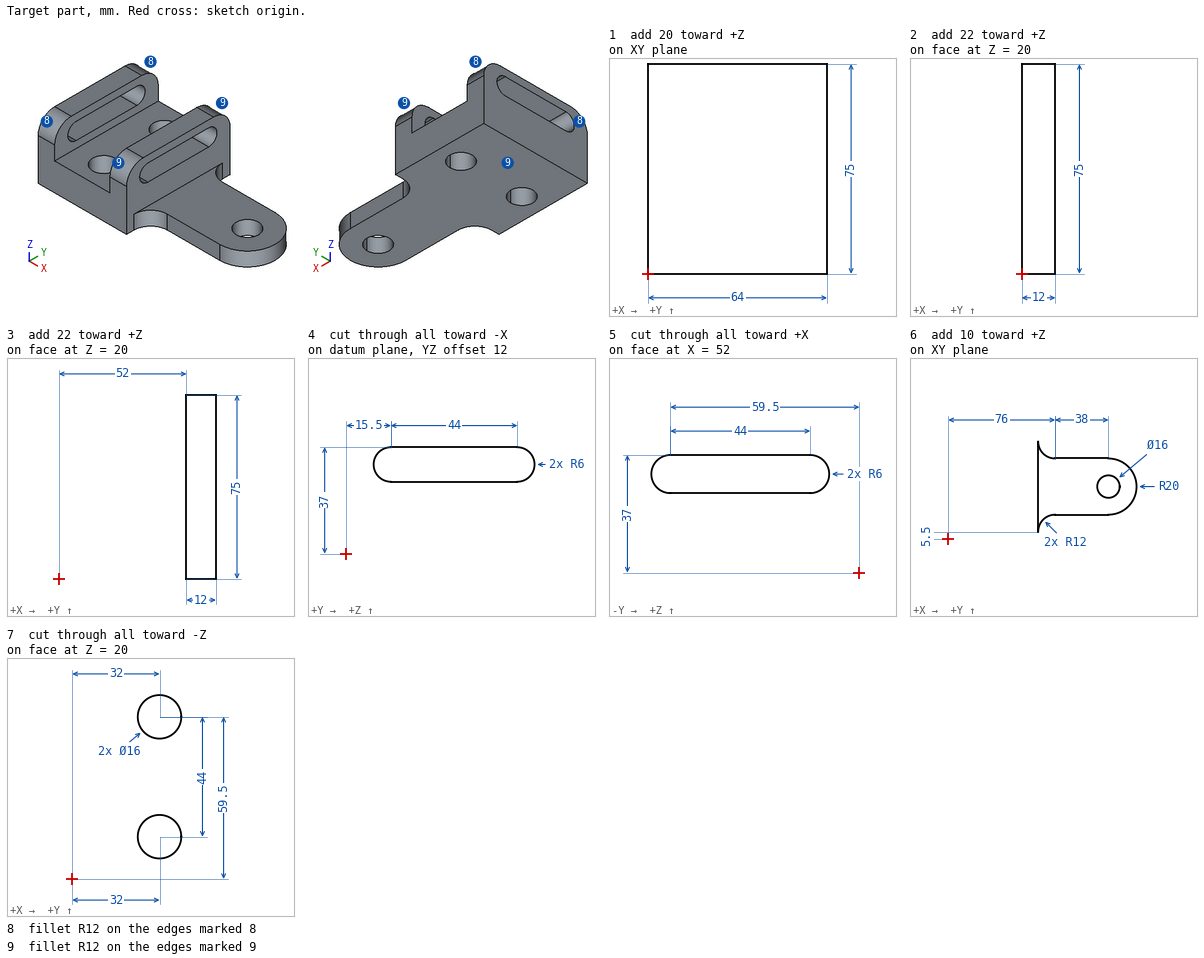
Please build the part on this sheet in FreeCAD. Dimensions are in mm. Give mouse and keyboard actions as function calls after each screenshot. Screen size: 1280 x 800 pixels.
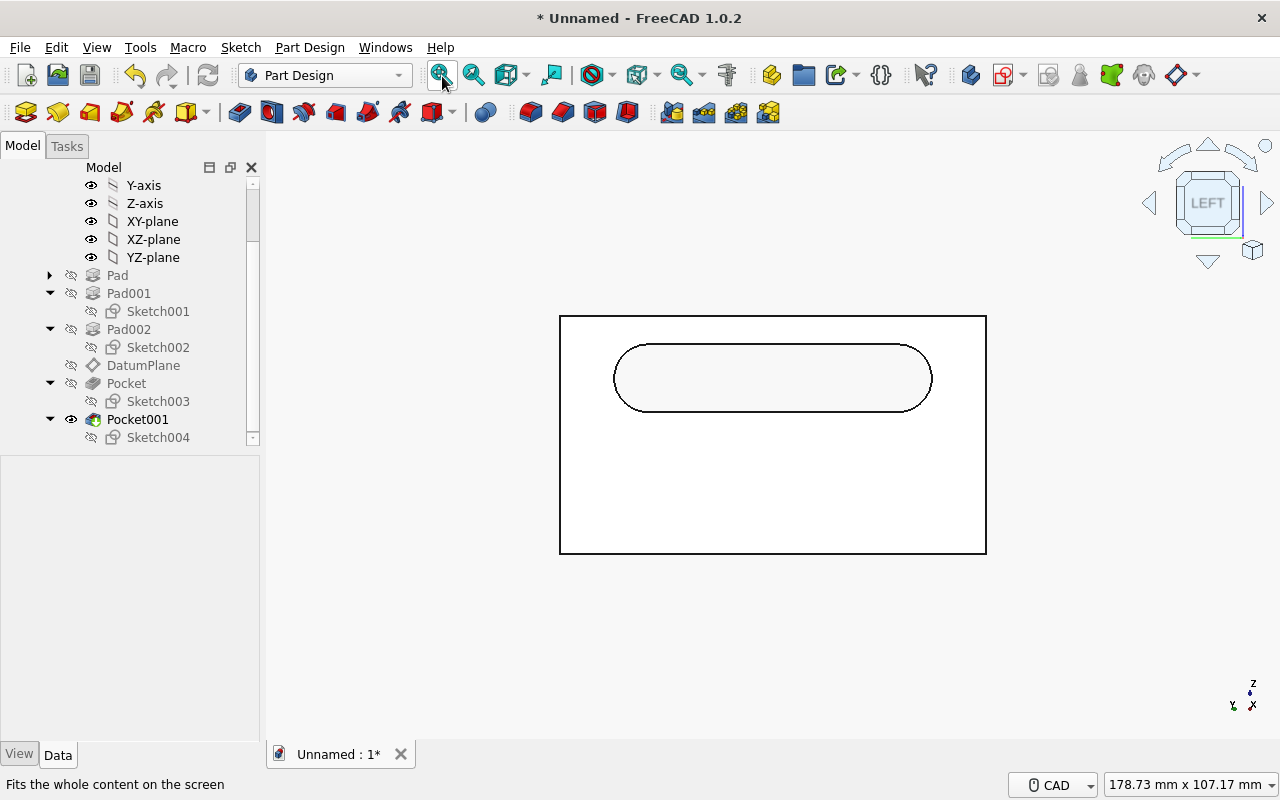
click(1004, 76)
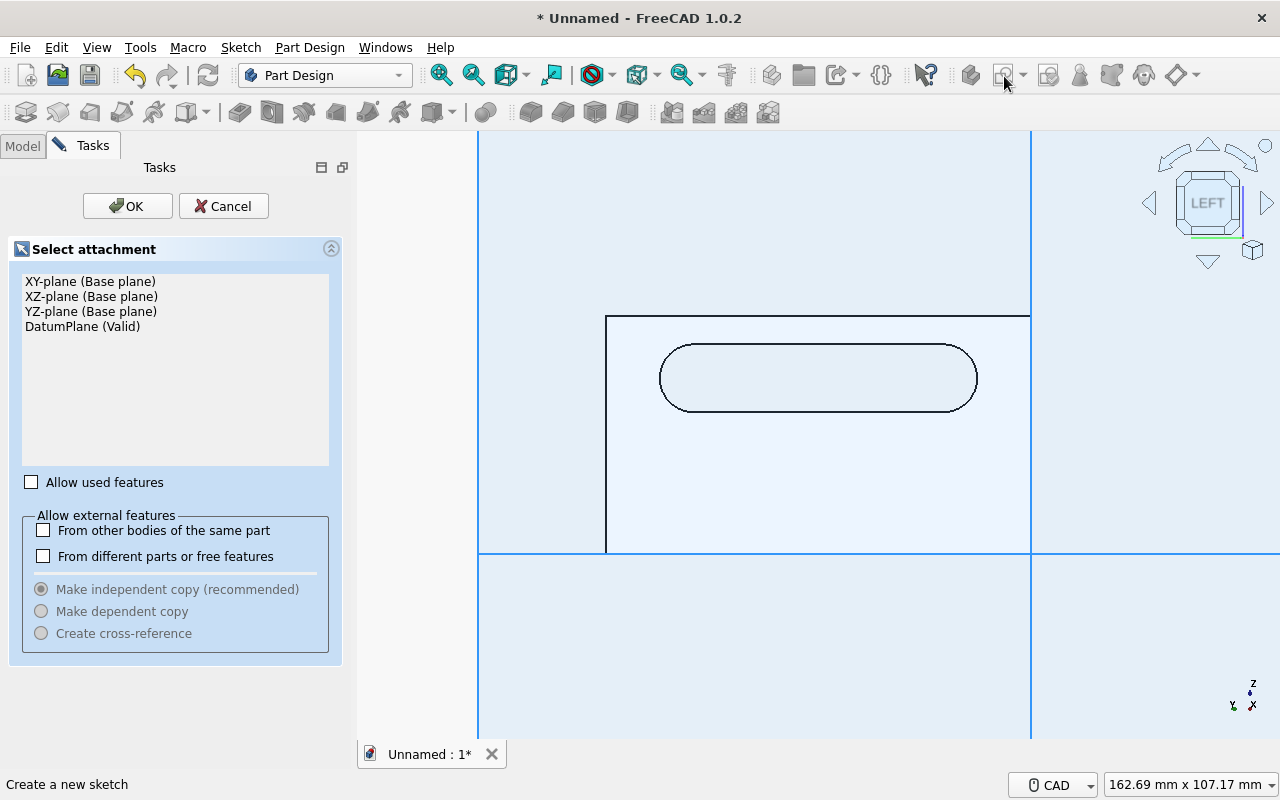
click(82, 282)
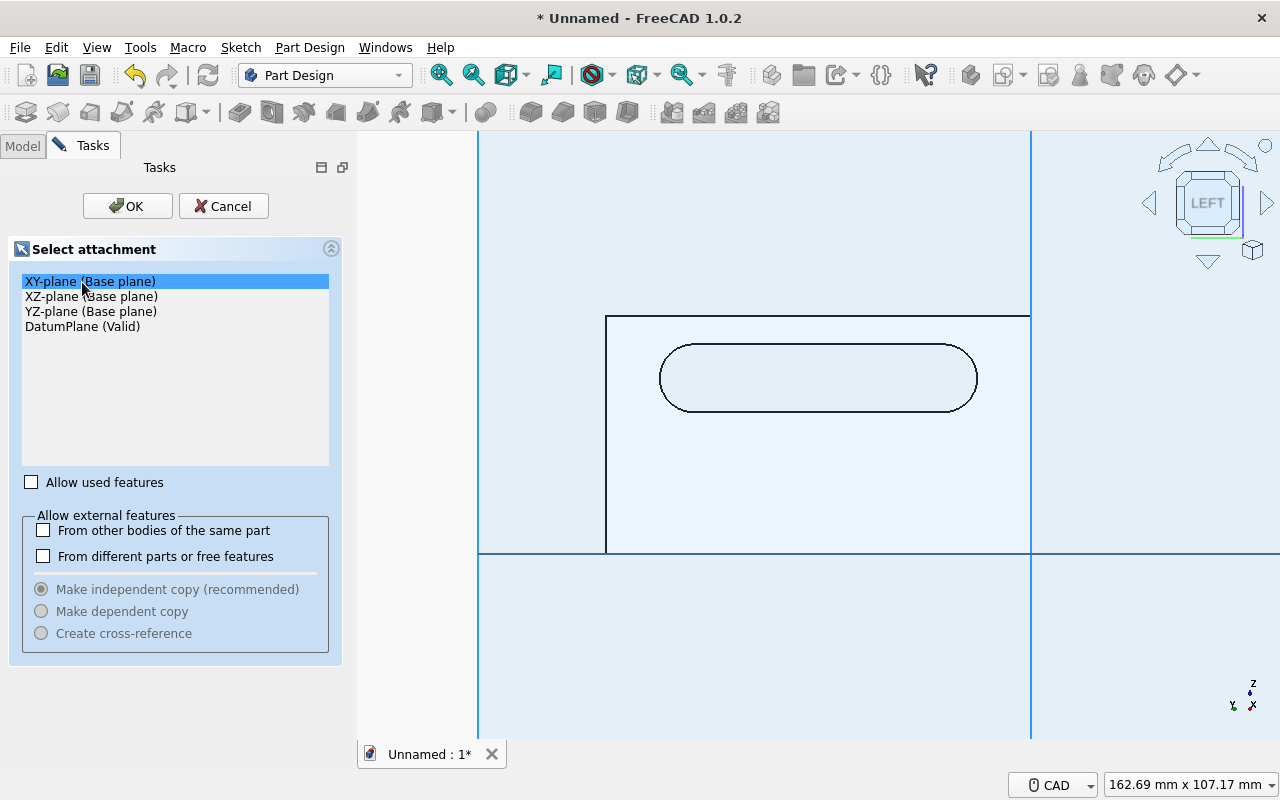
click(128, 206)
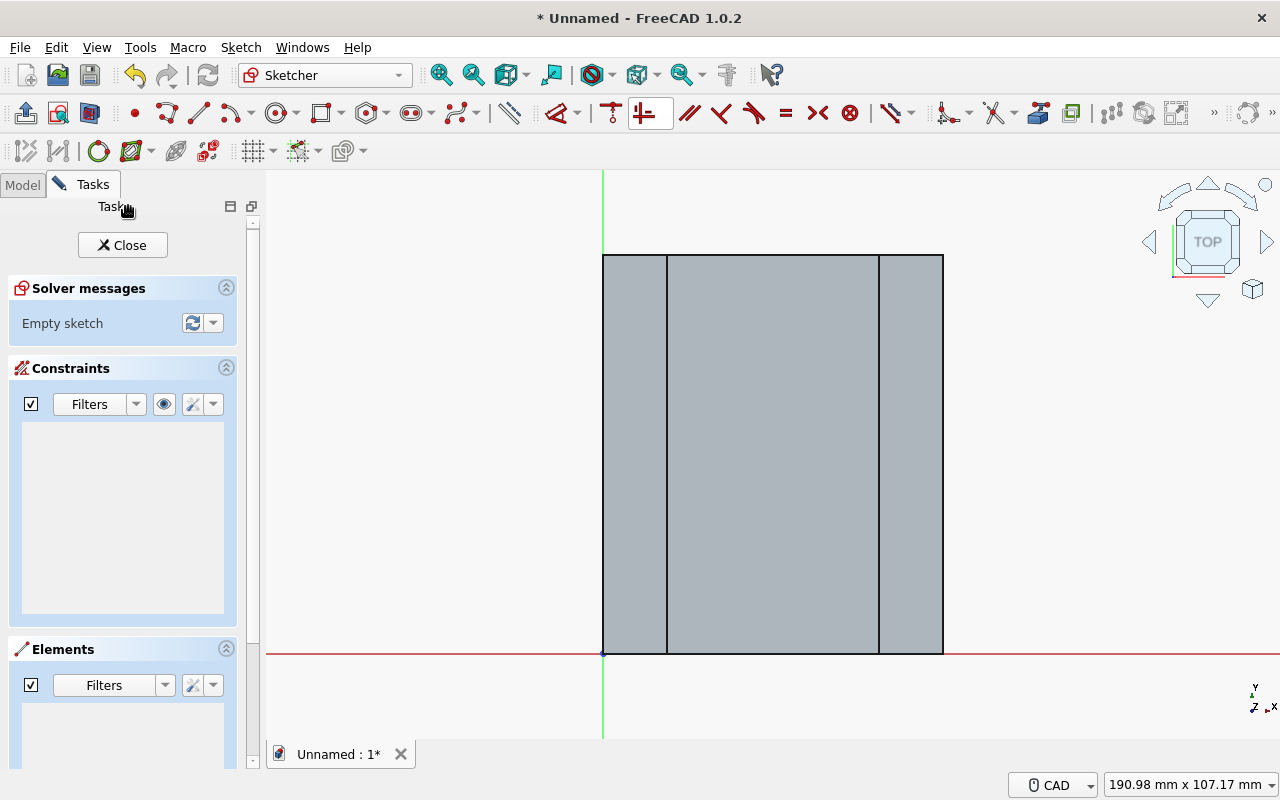
click(90, 114)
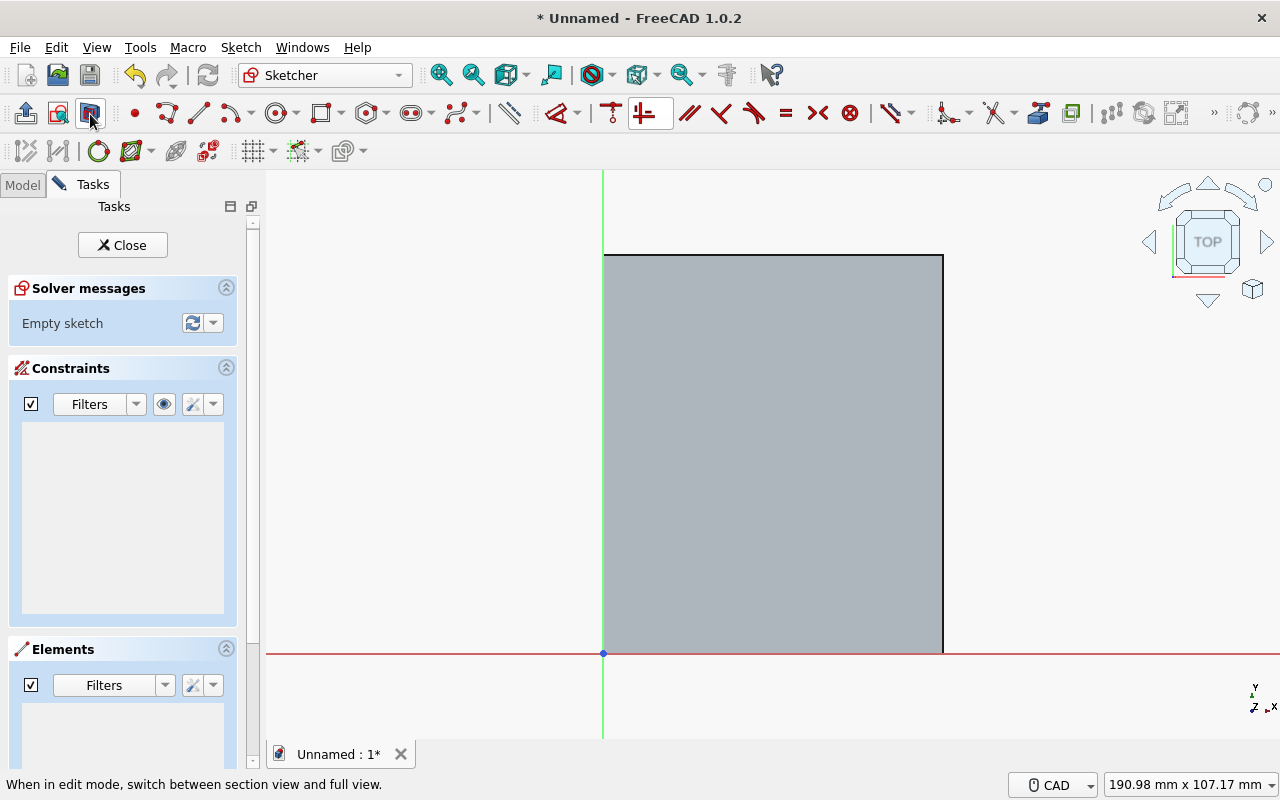
scroll(294, 425, down, 2)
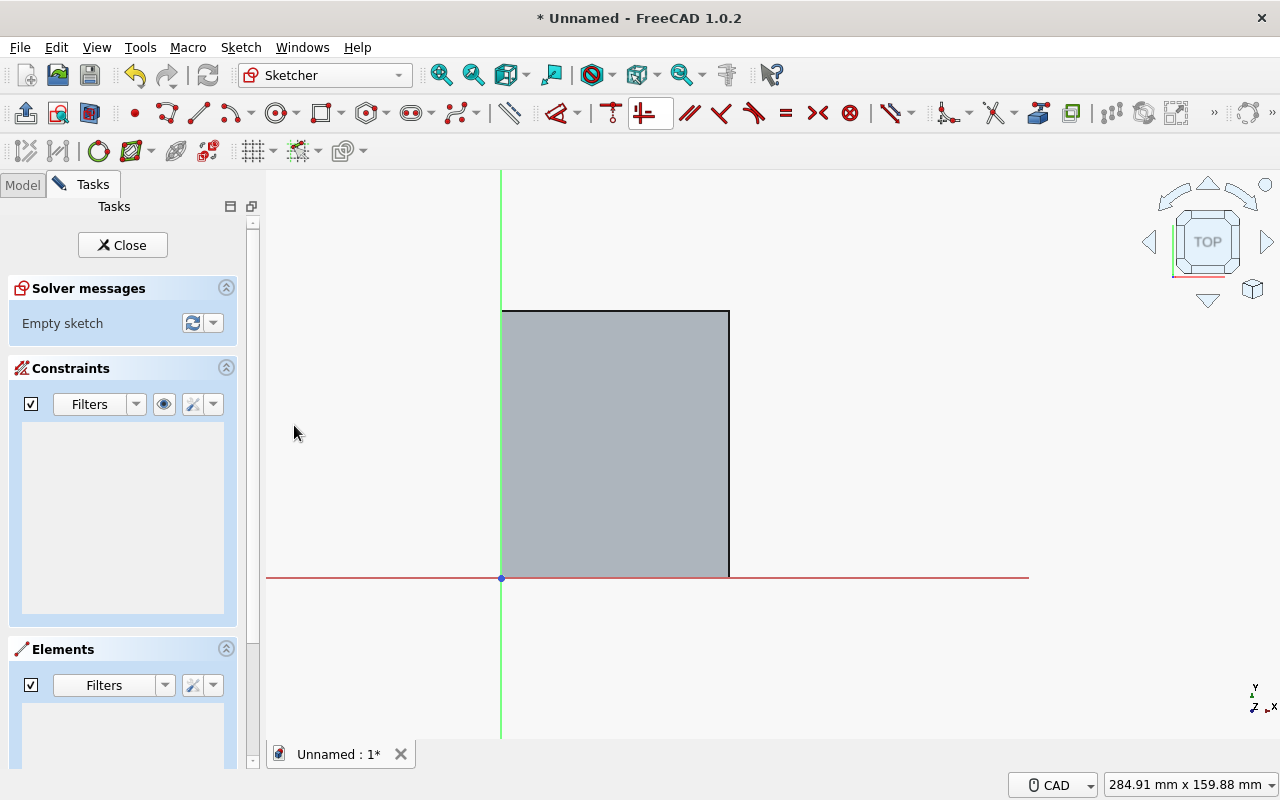
click(200, 114)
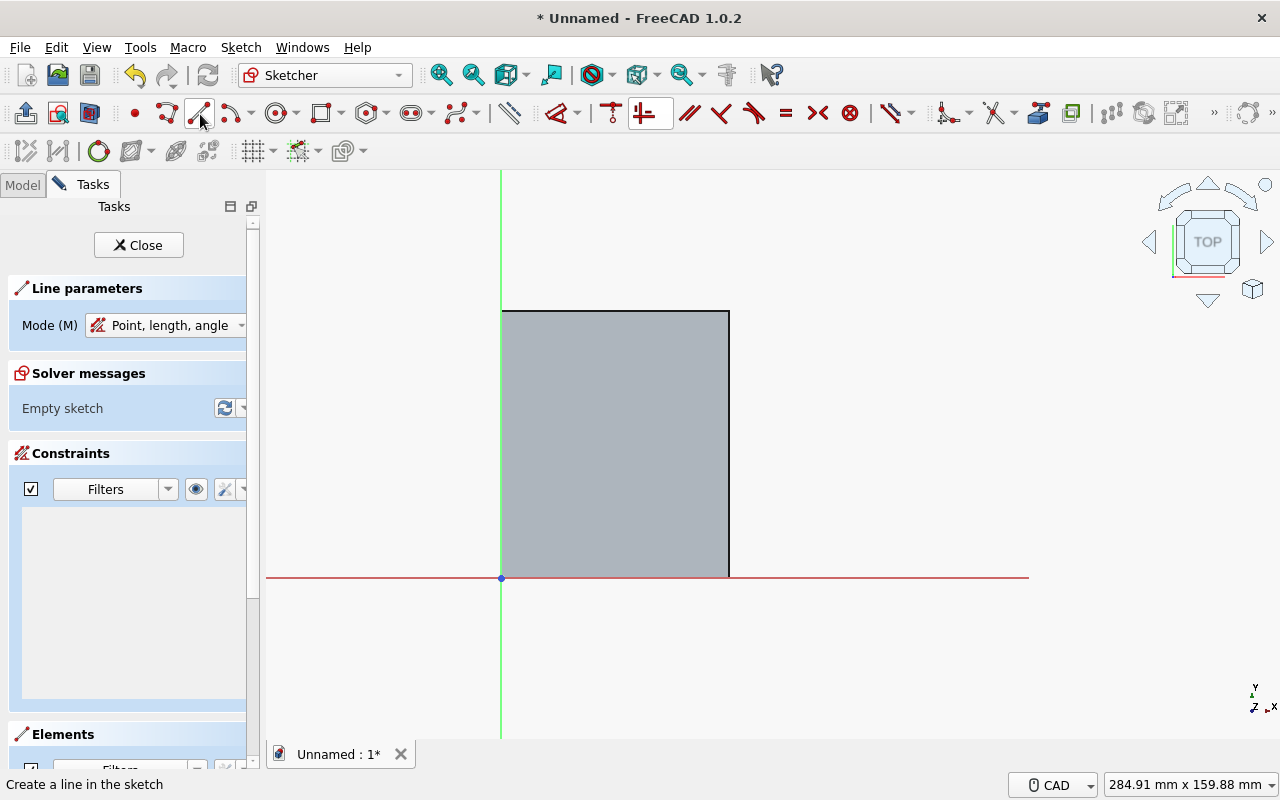
click(907, 374)
click(772, 374)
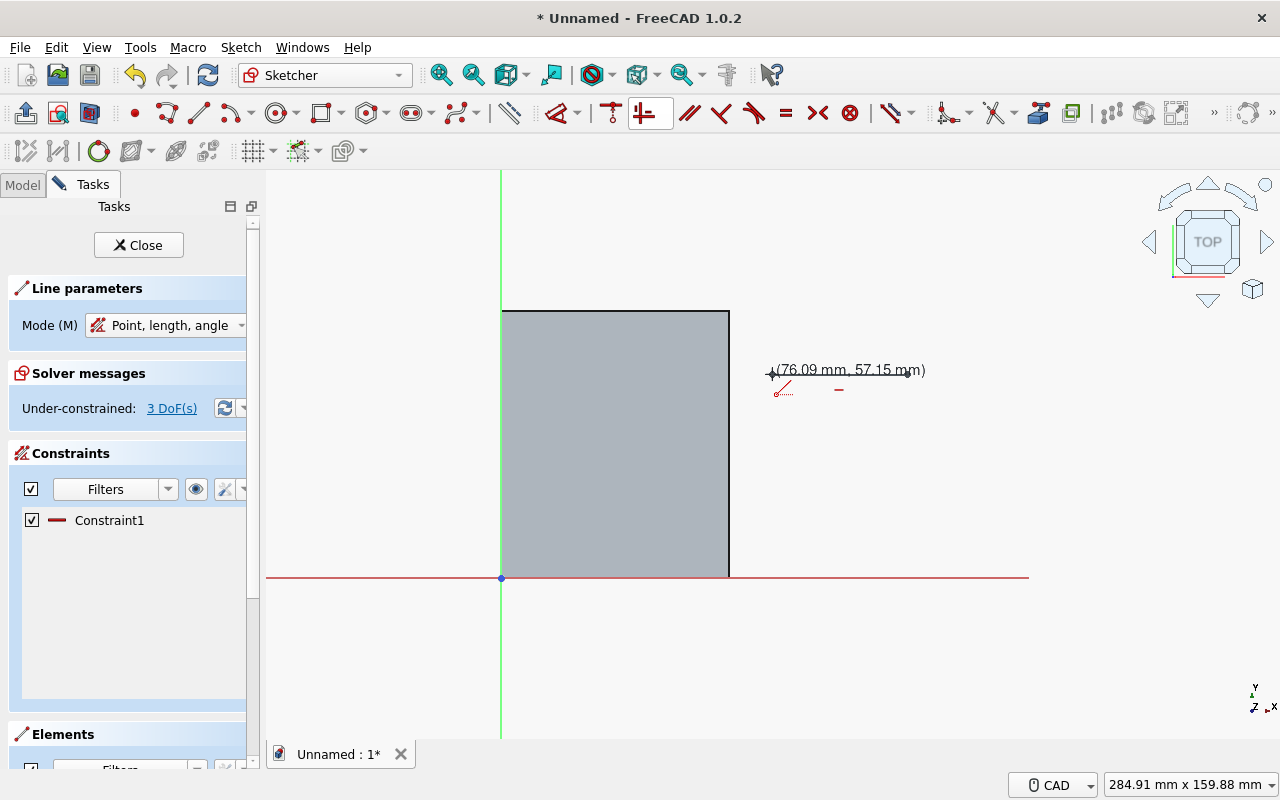
click(729, 331)
click(729, 559)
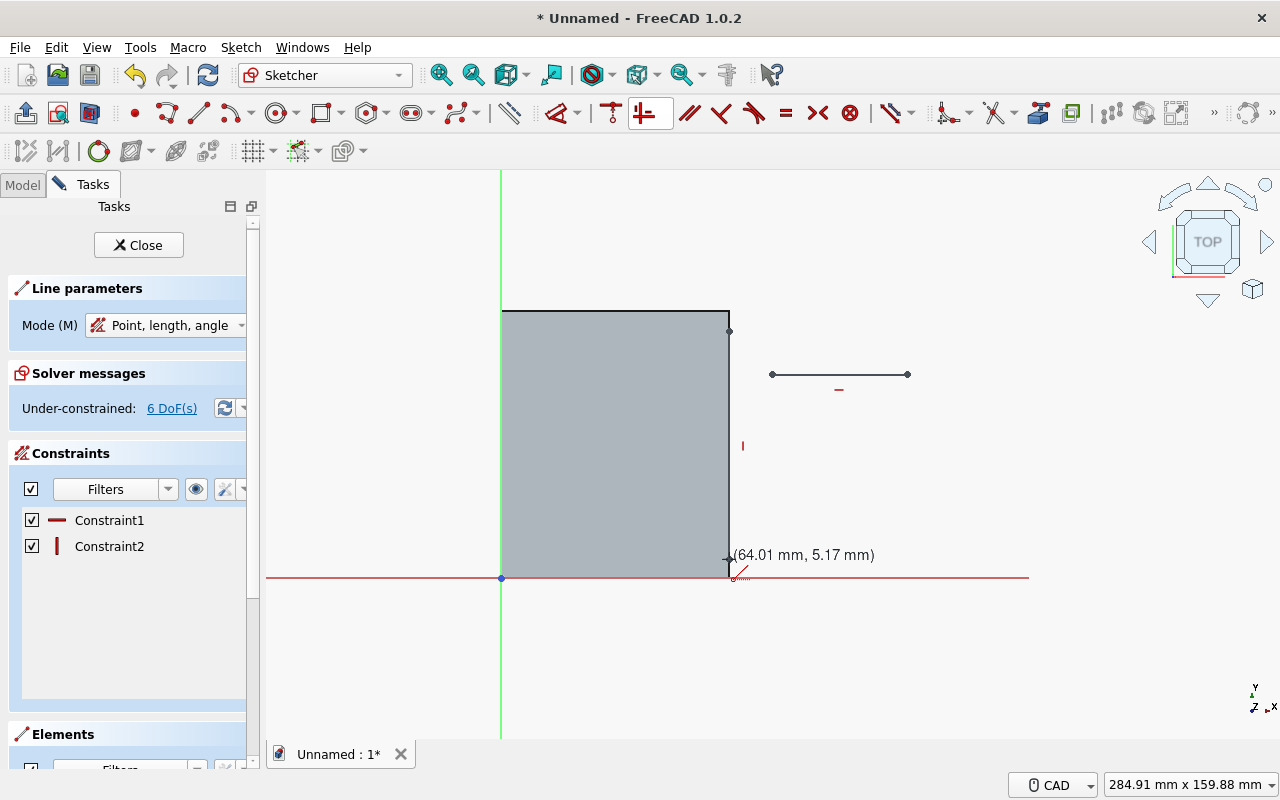
click(772, 516)
click(907, 516)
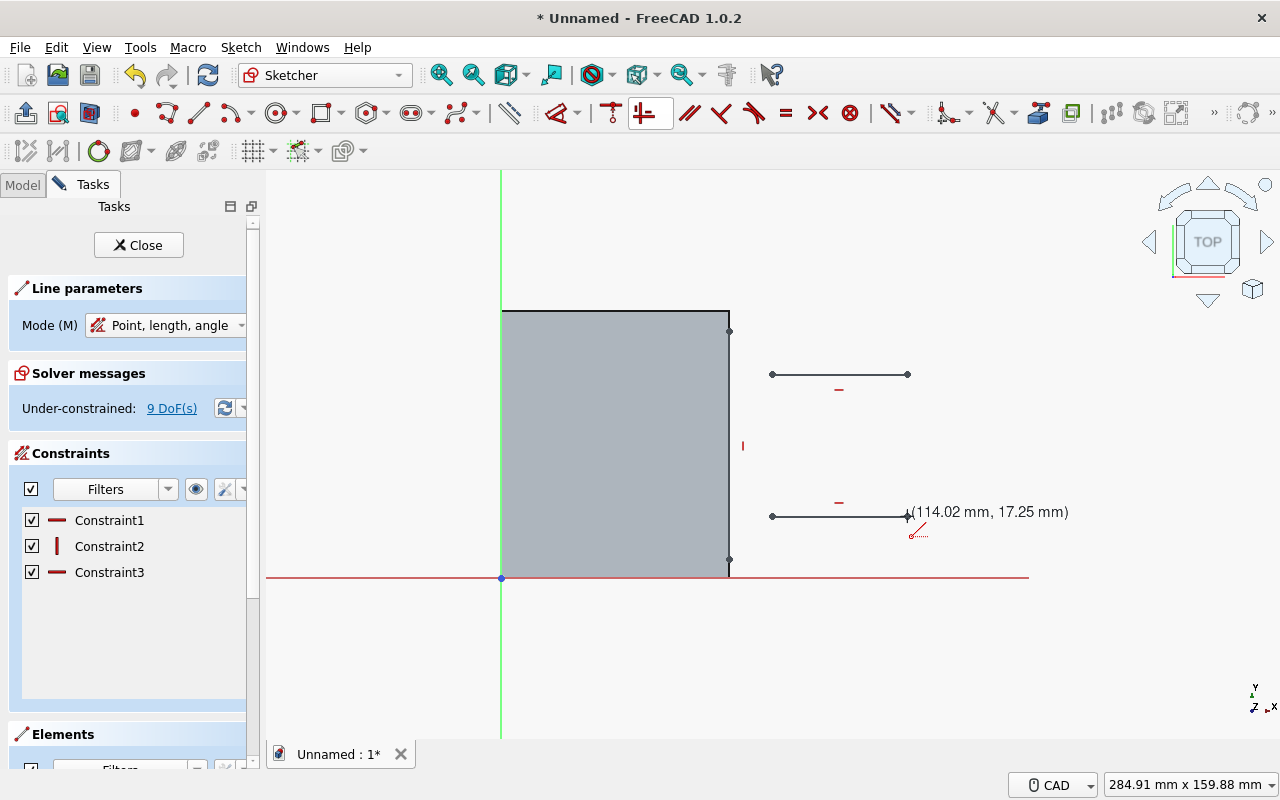
key(g)
key(3)
key(a)